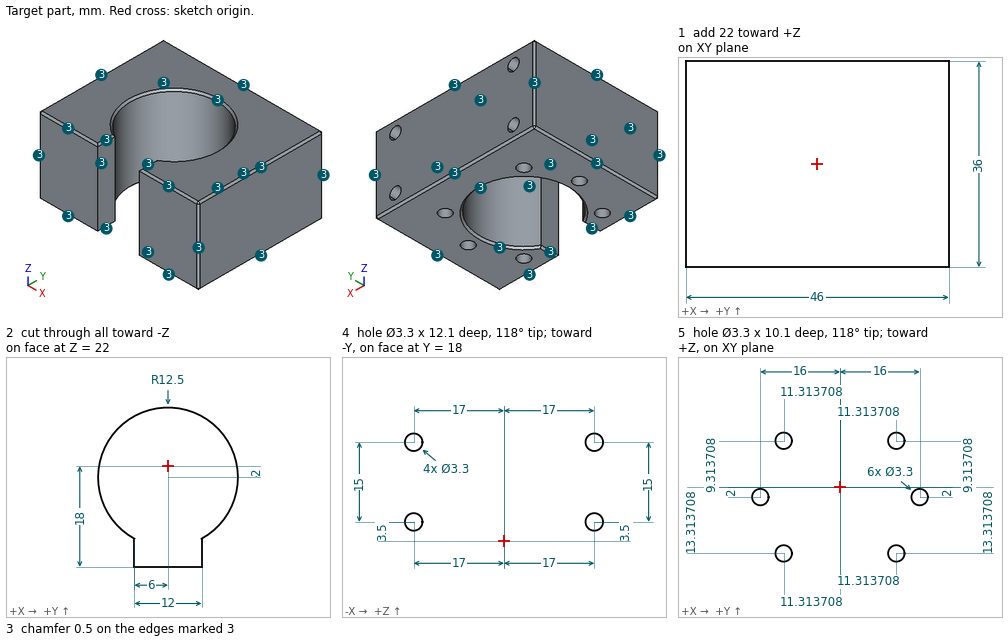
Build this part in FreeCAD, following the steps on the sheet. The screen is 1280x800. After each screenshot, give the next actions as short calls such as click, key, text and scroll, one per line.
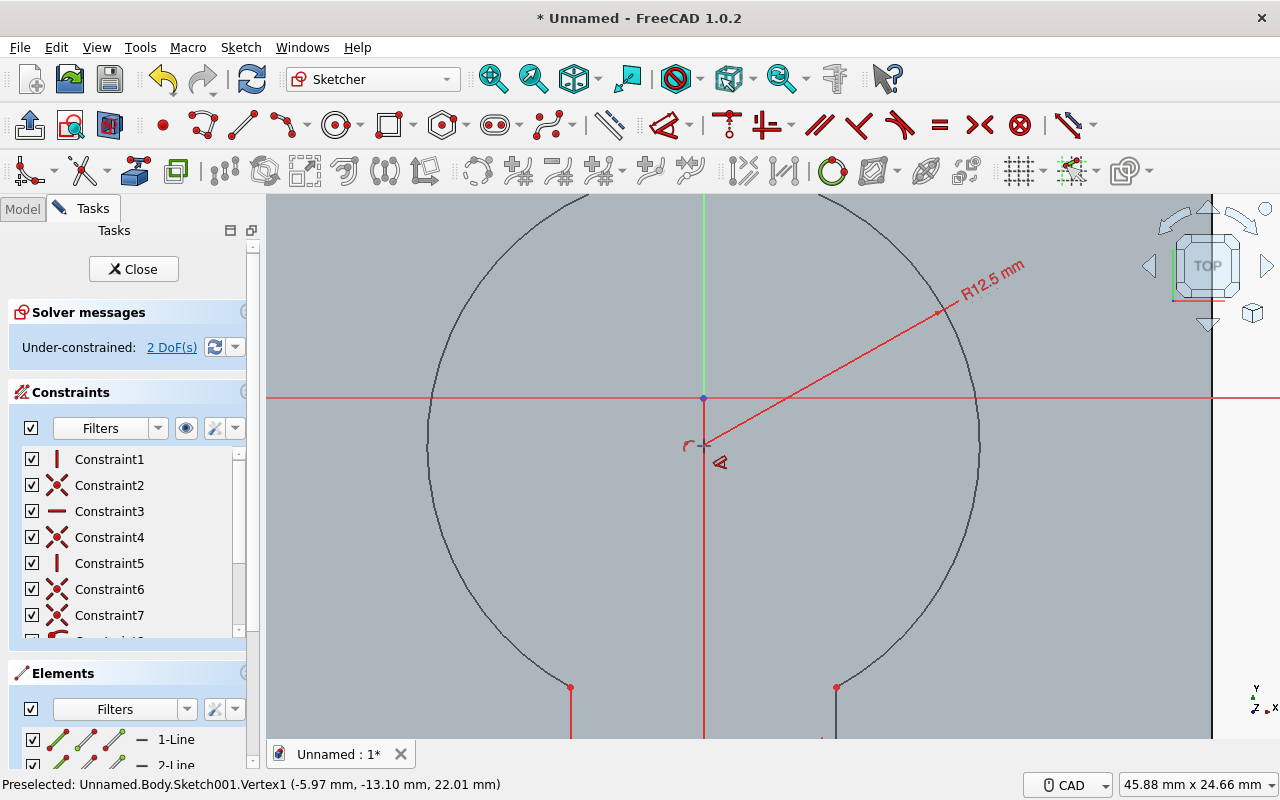
click(704, 445)
click(738, 422)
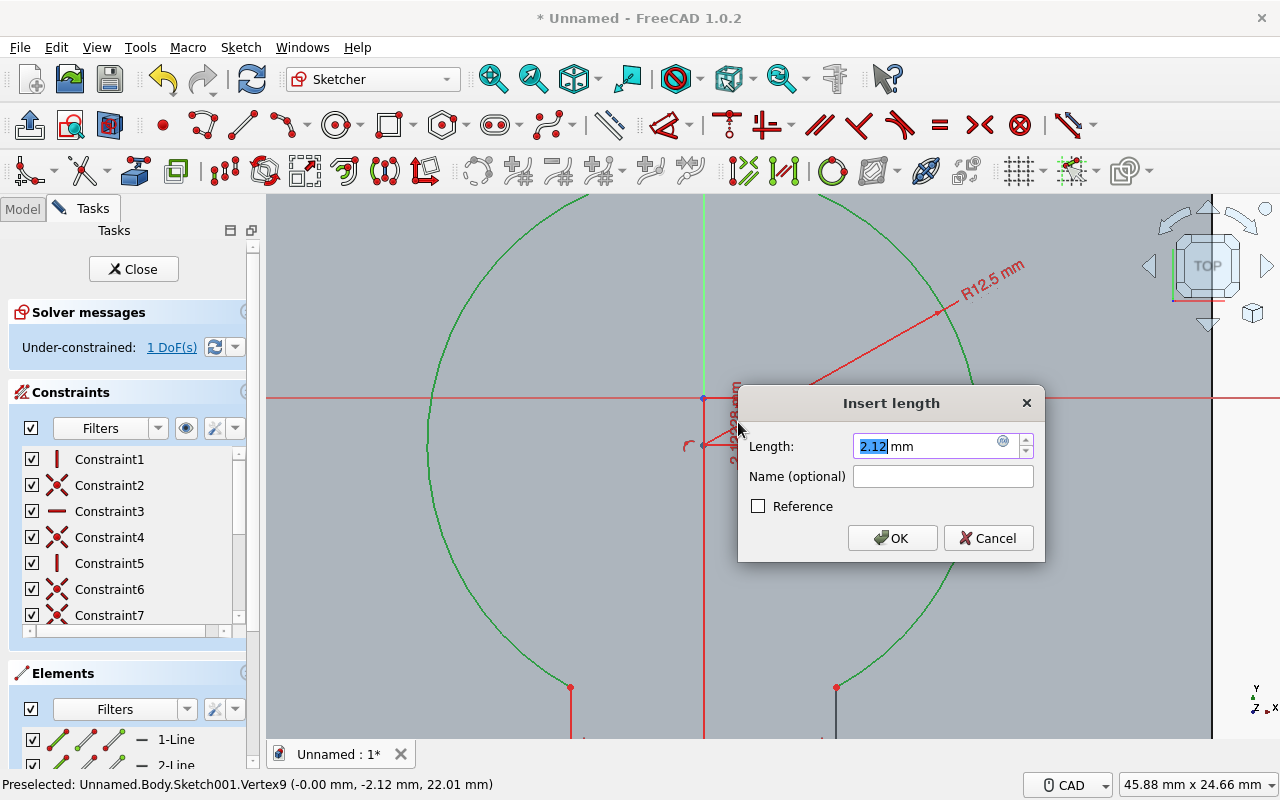
text(2)
key(Return)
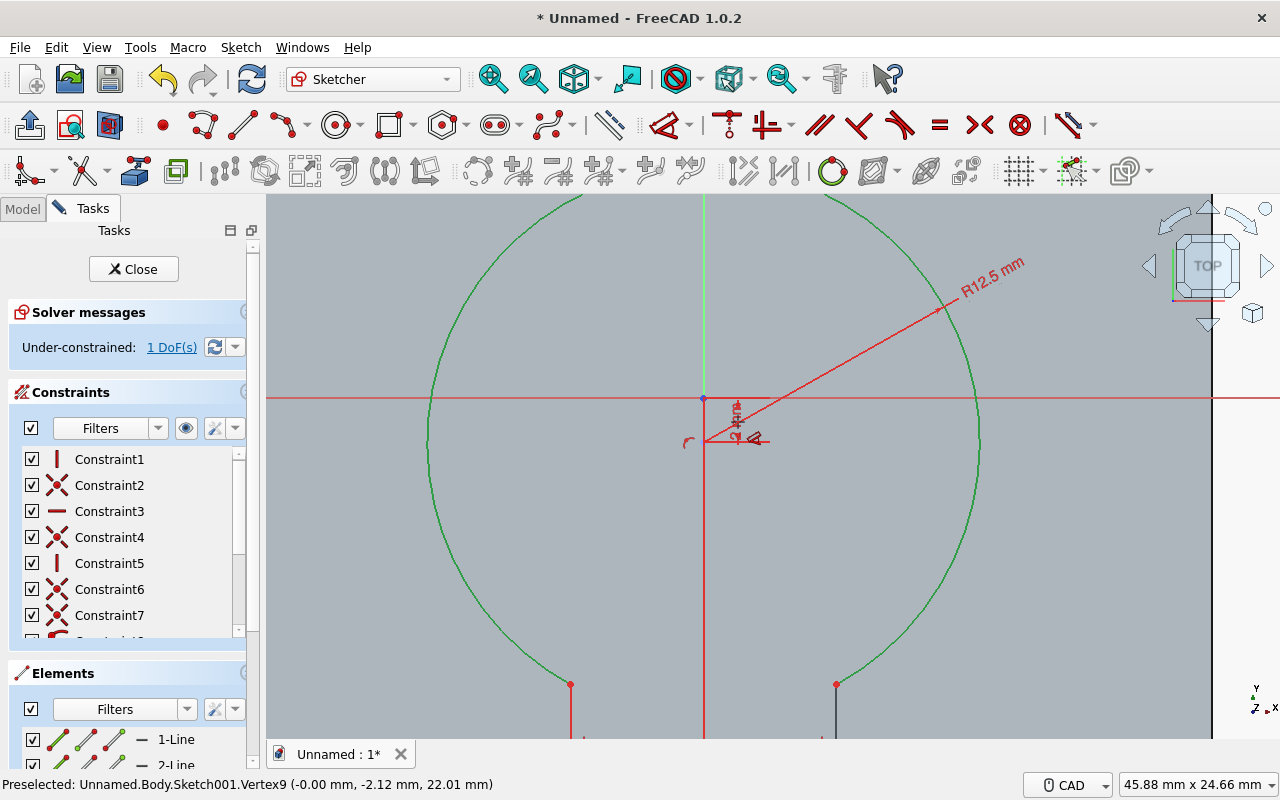
scroll(706, 449, down, 3)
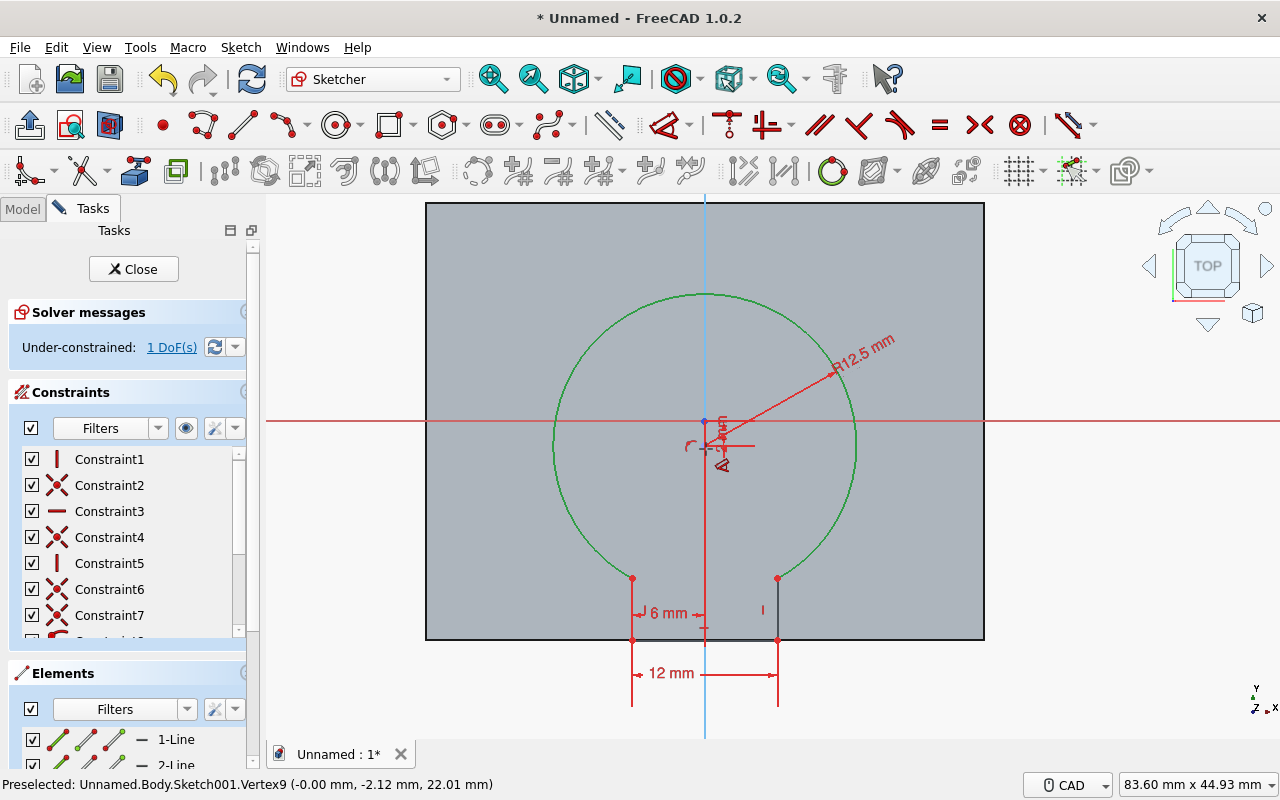
click(632, 641)
click(598, 531)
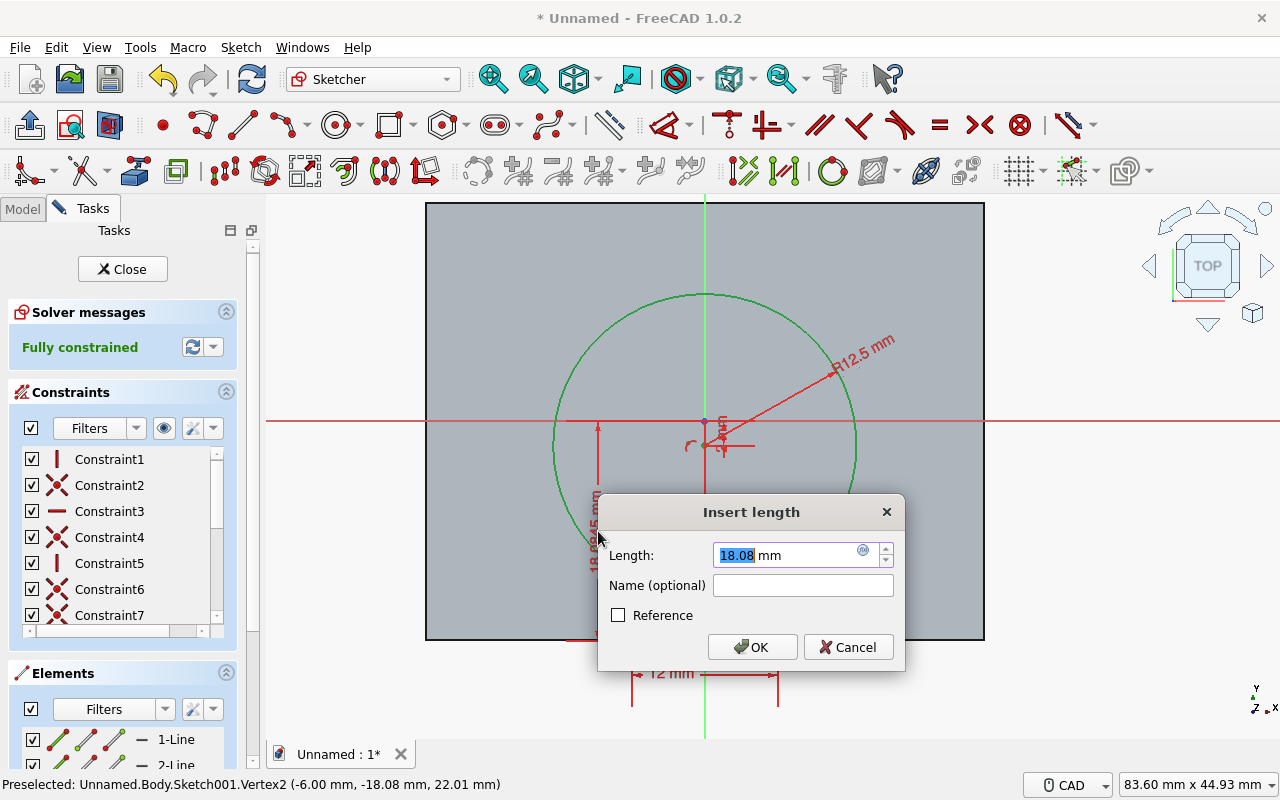
text(18)
key(Return)
key(Escape)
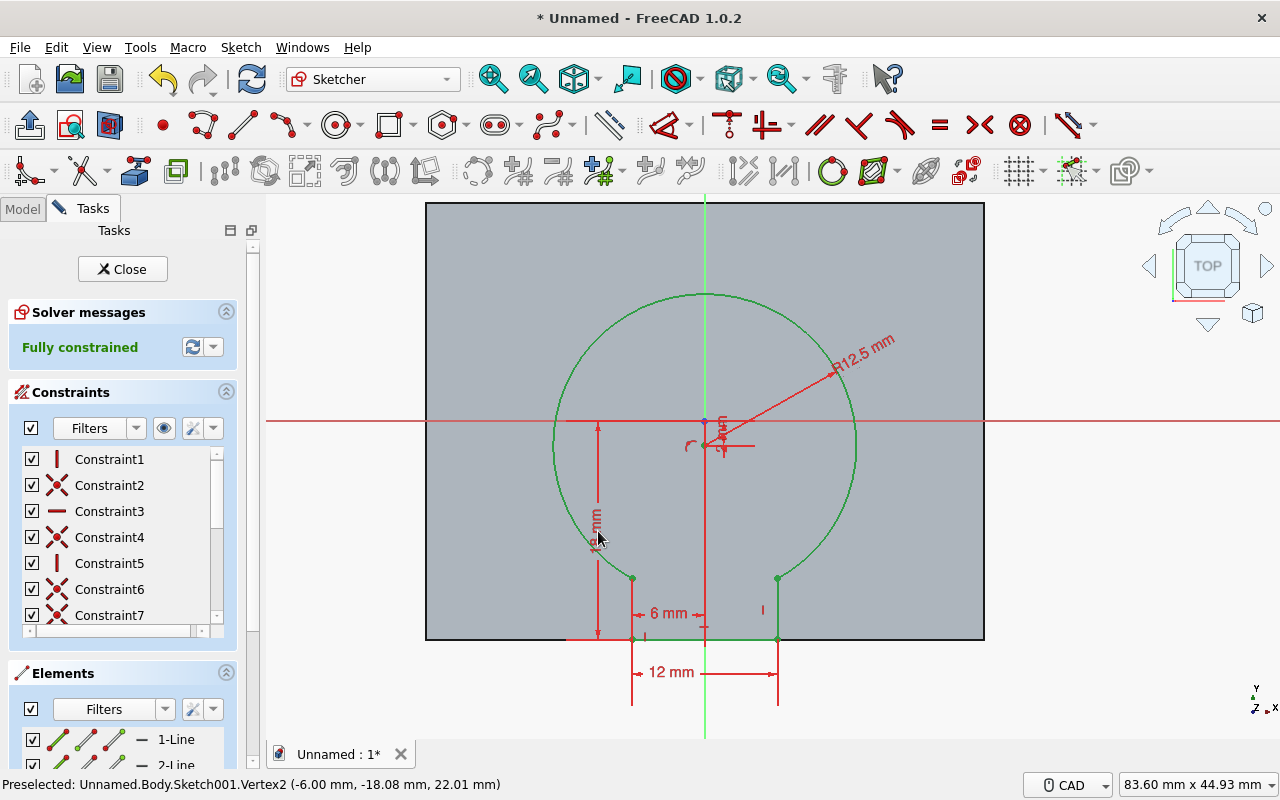
click(123, 269)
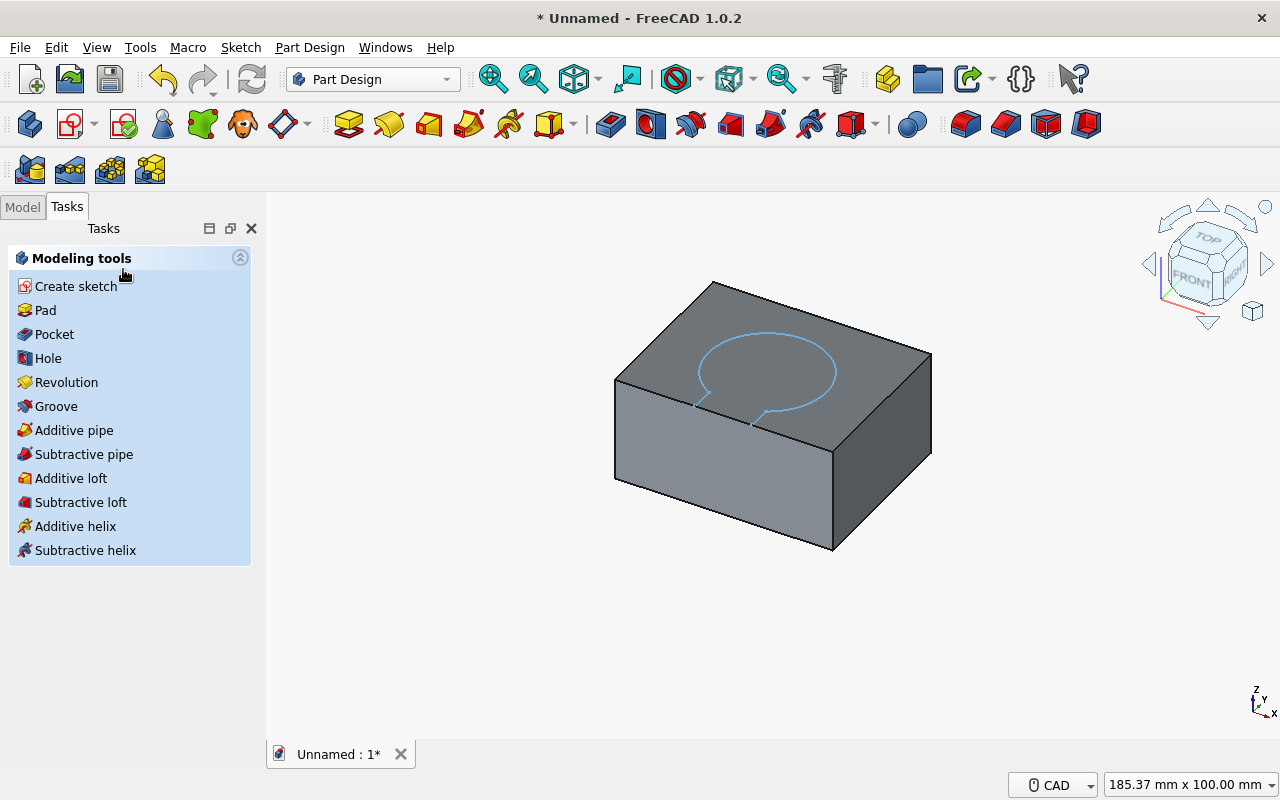
click(612, 124)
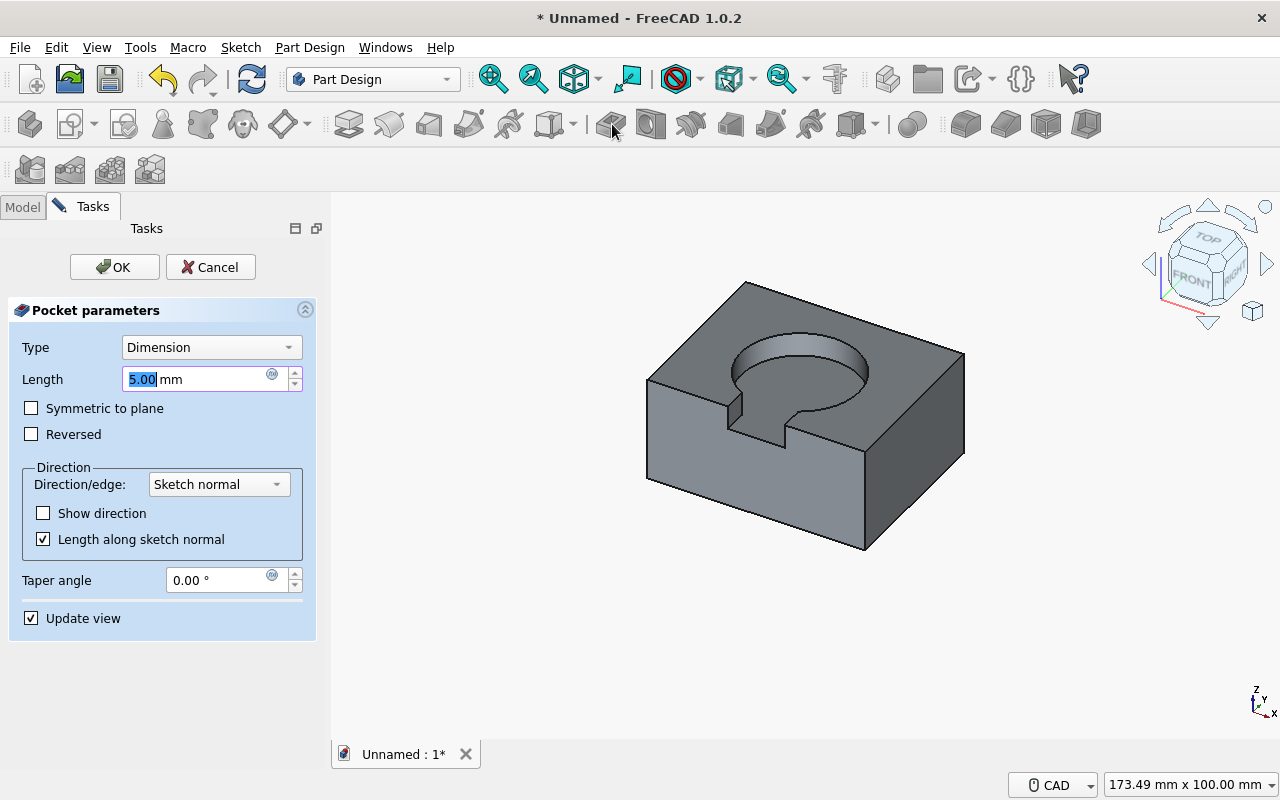
click(212, 348)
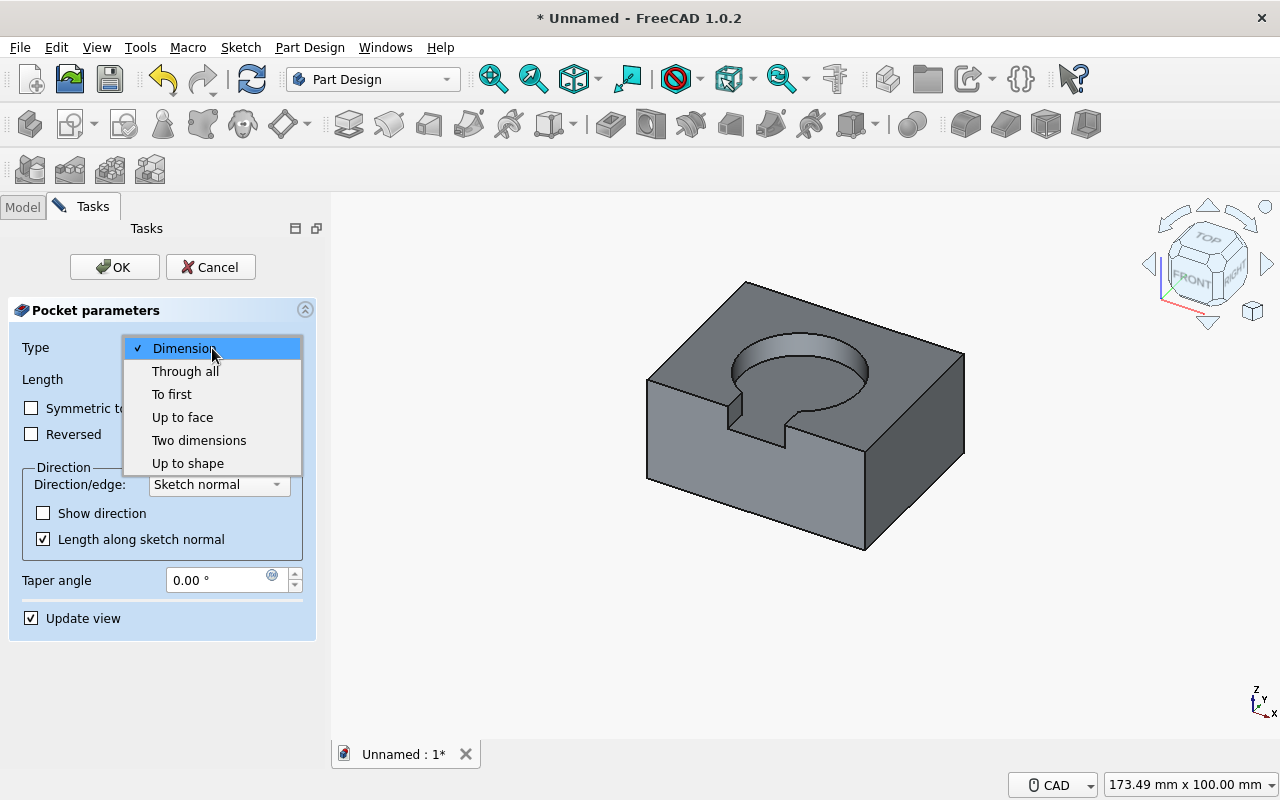
click(212, 372)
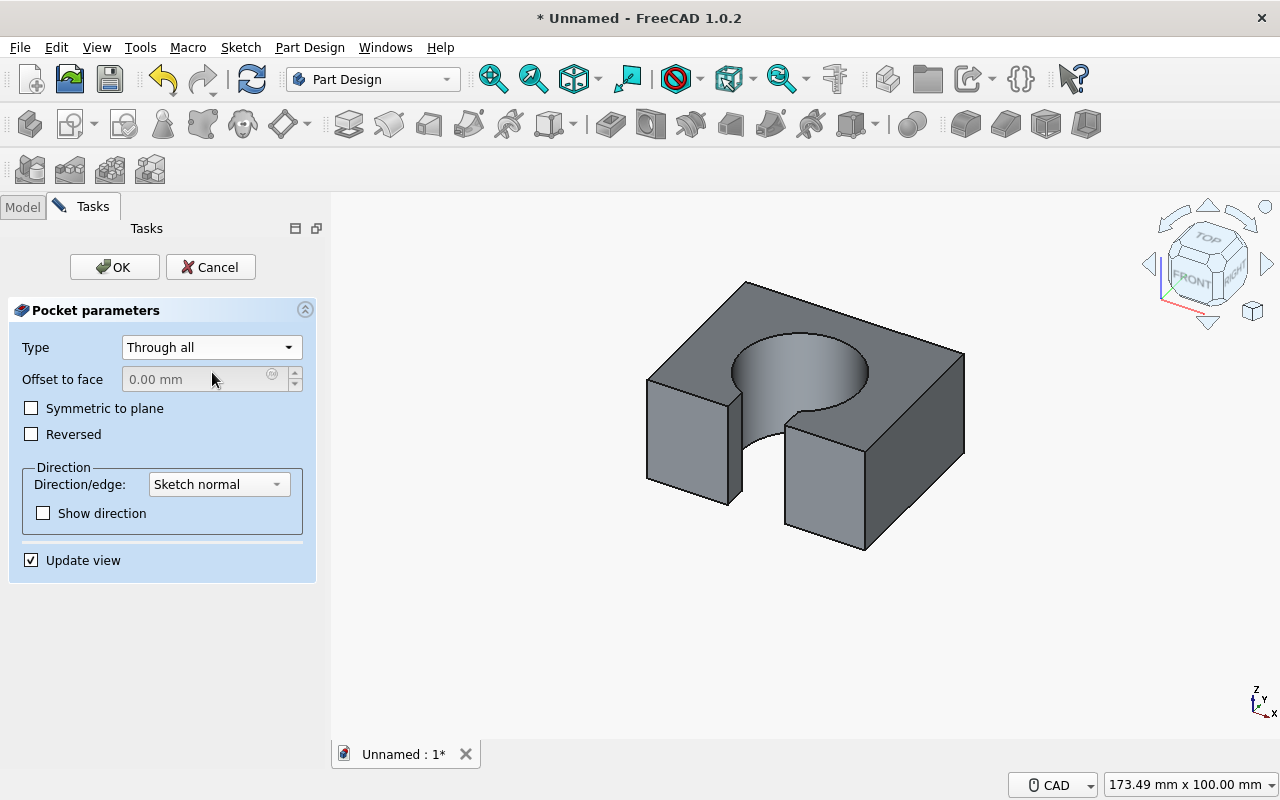
click(115, 267)